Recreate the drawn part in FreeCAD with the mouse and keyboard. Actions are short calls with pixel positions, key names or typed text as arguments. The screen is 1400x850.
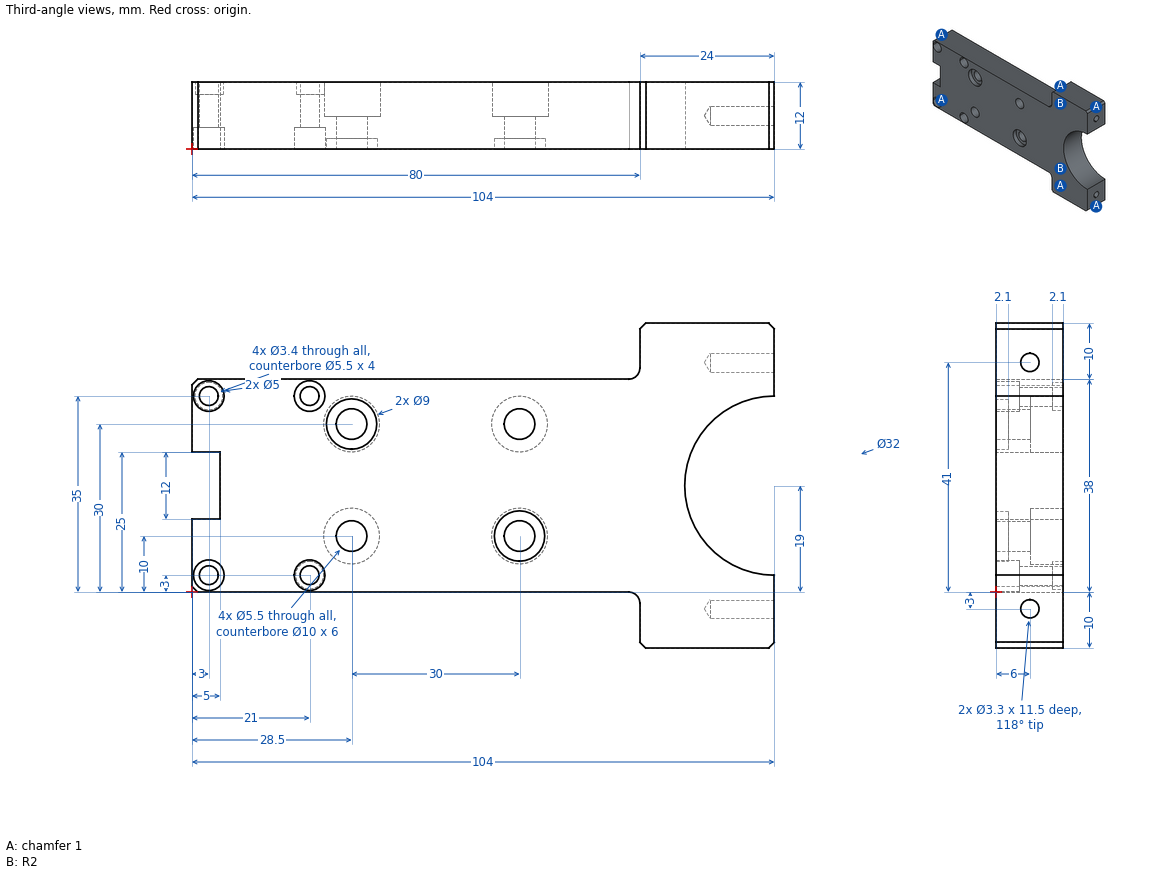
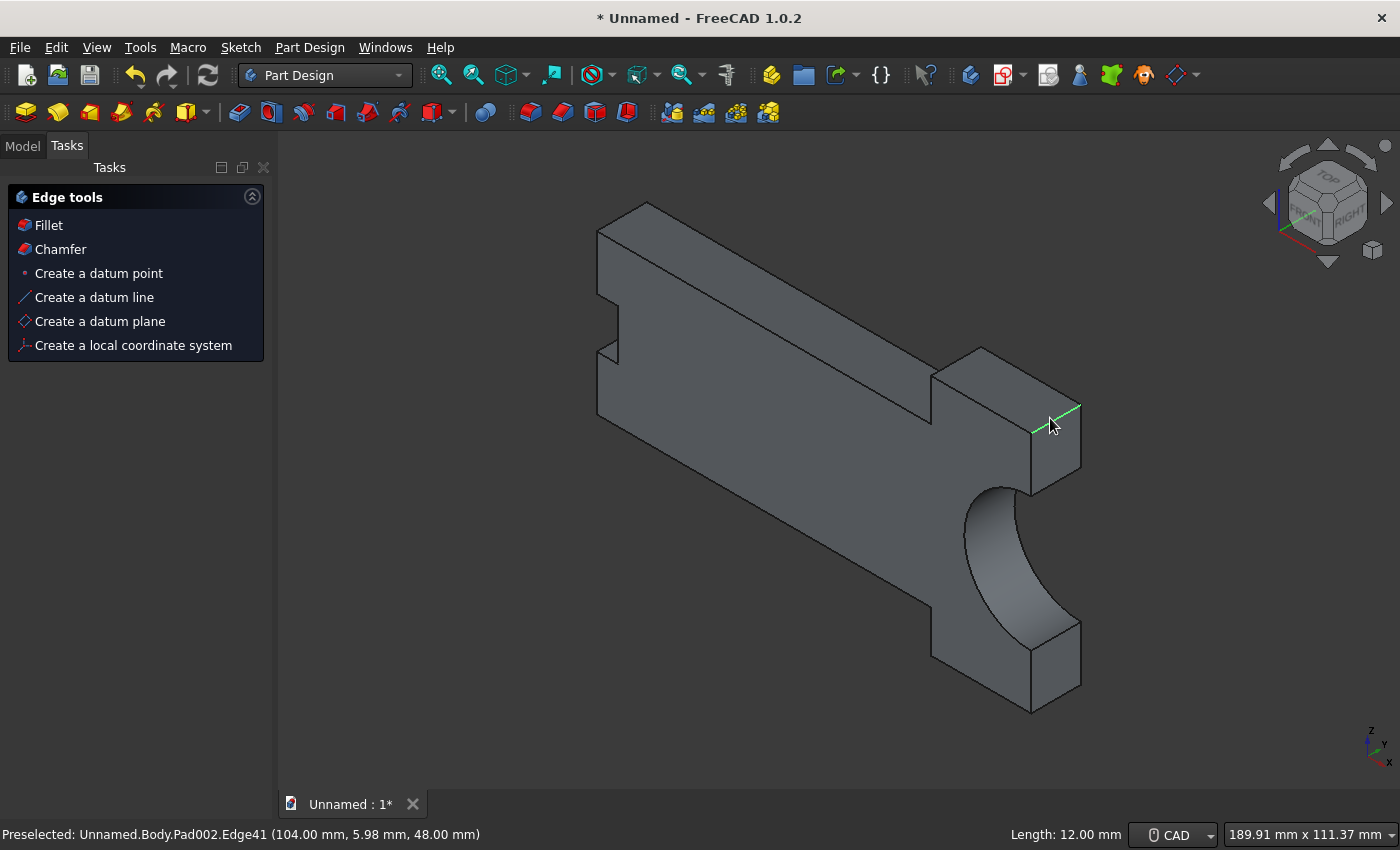
key(2)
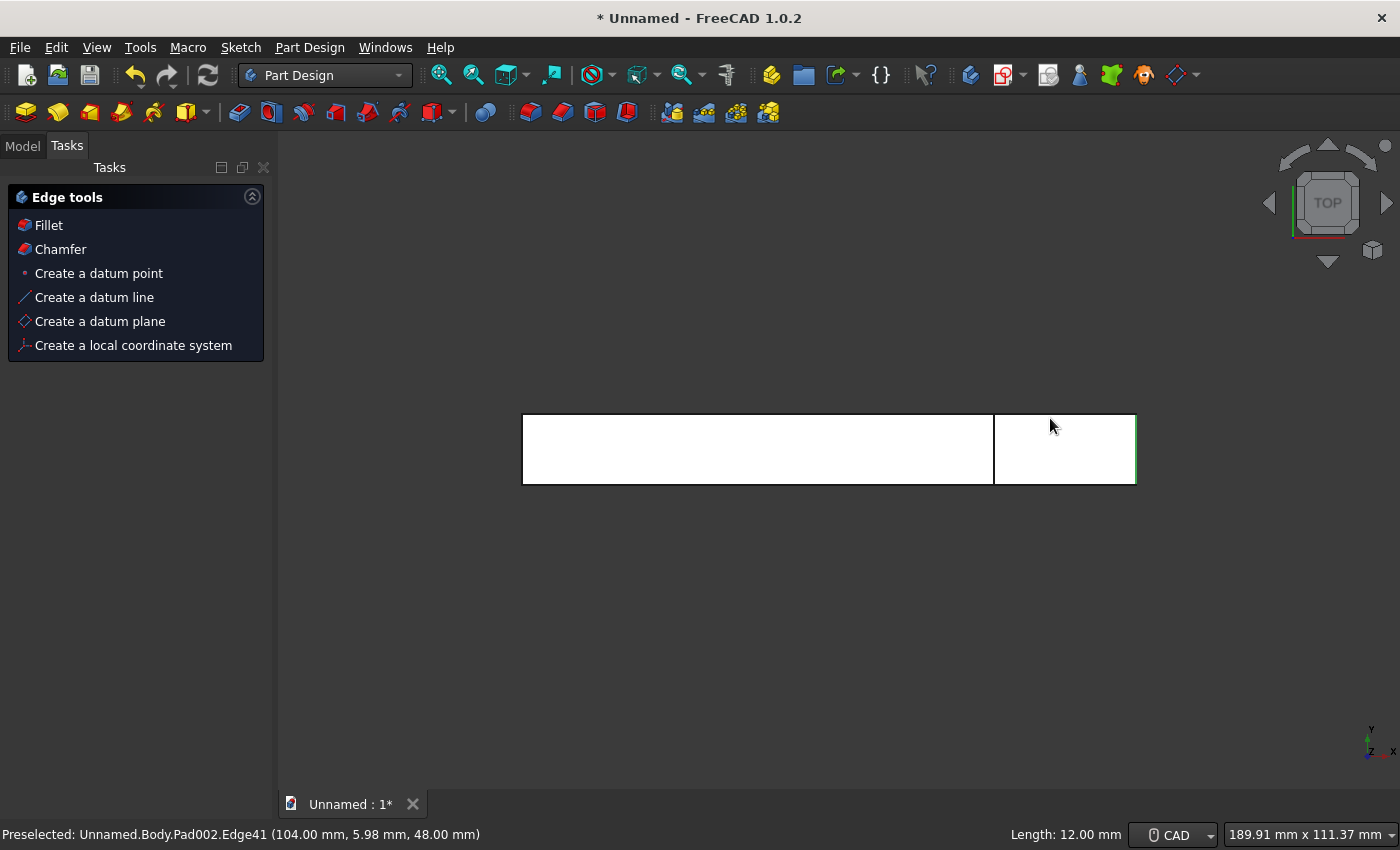
click(522, 449, ctrl)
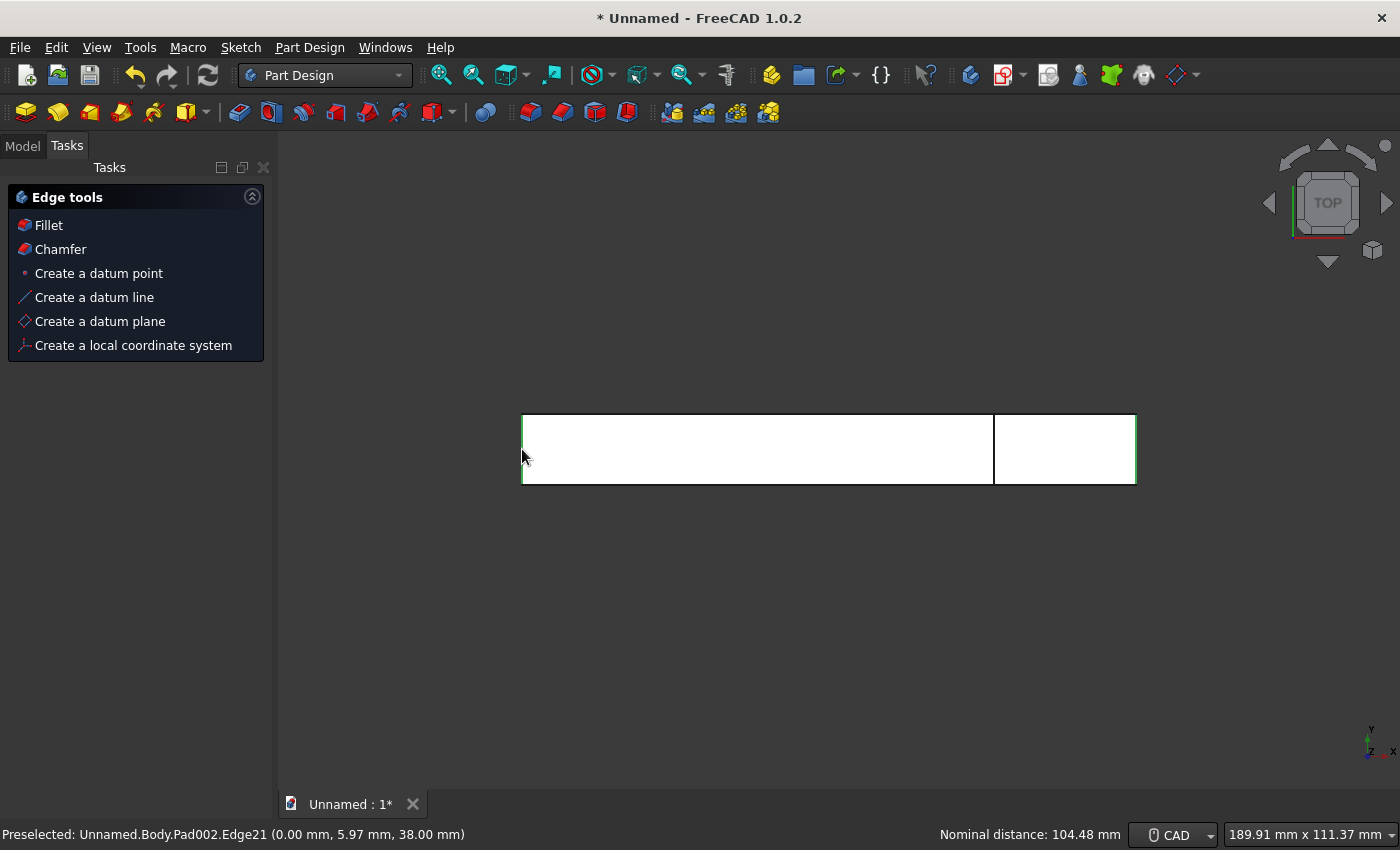
click(994, 449, ctrl)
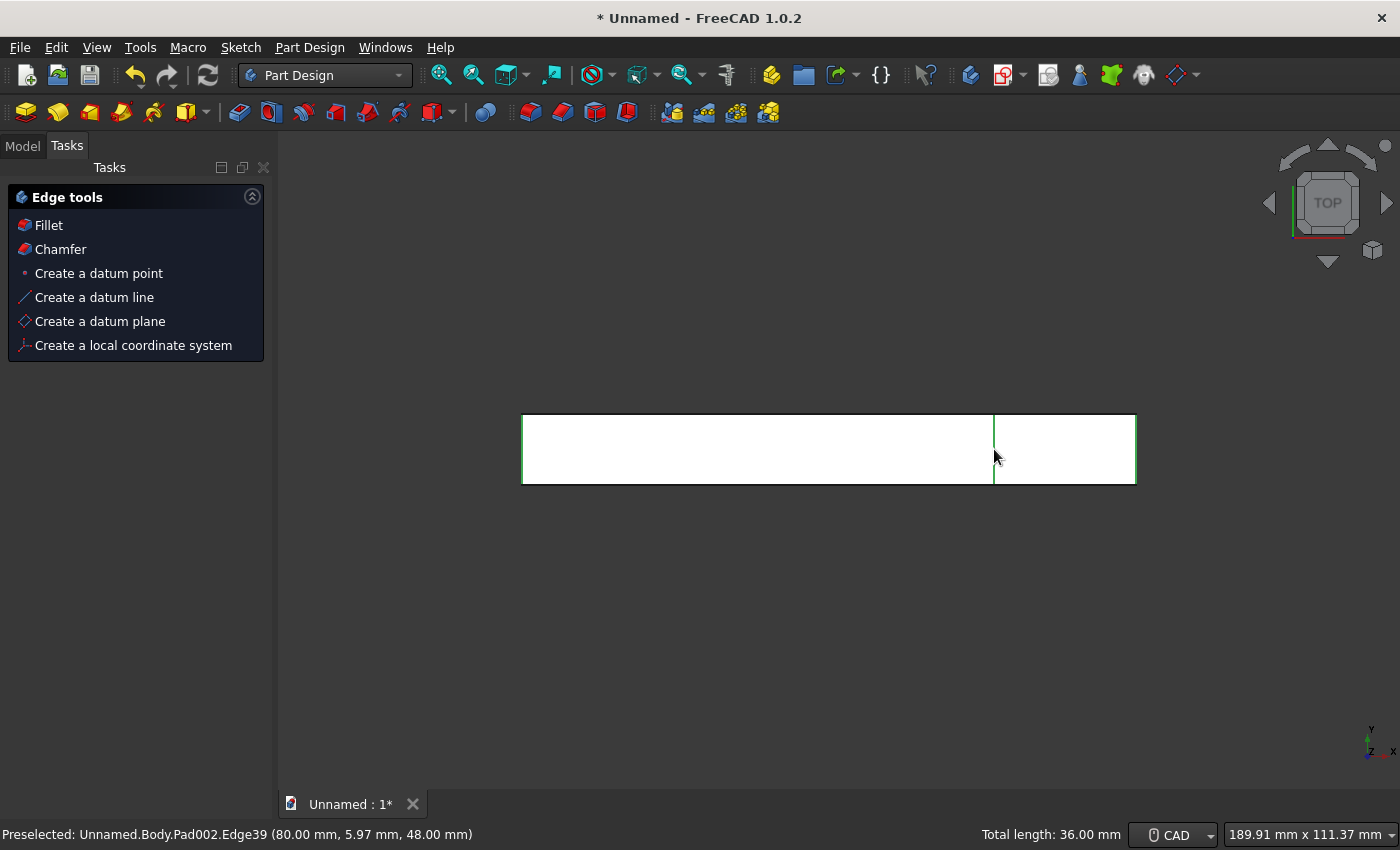
key(0)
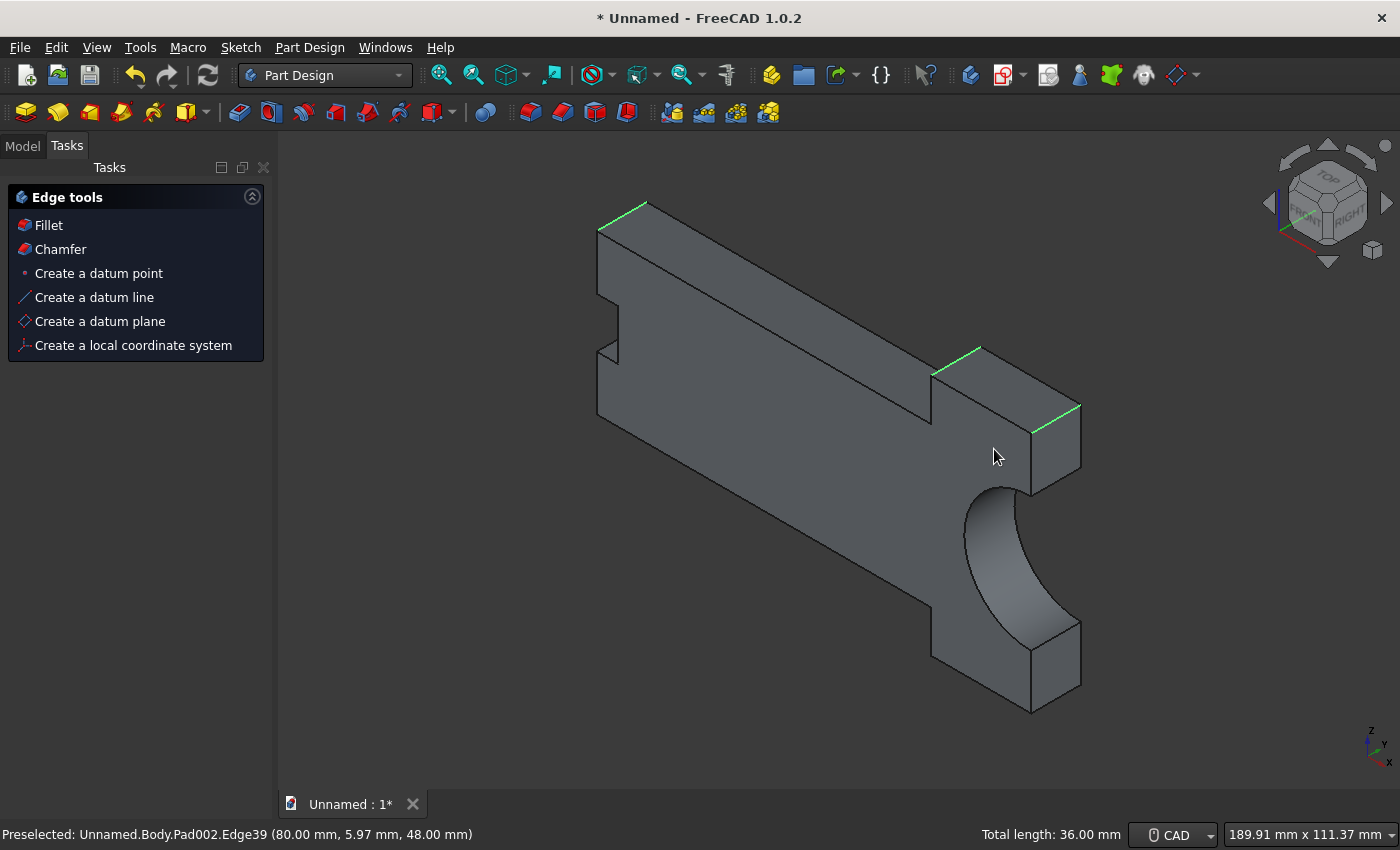
key(1)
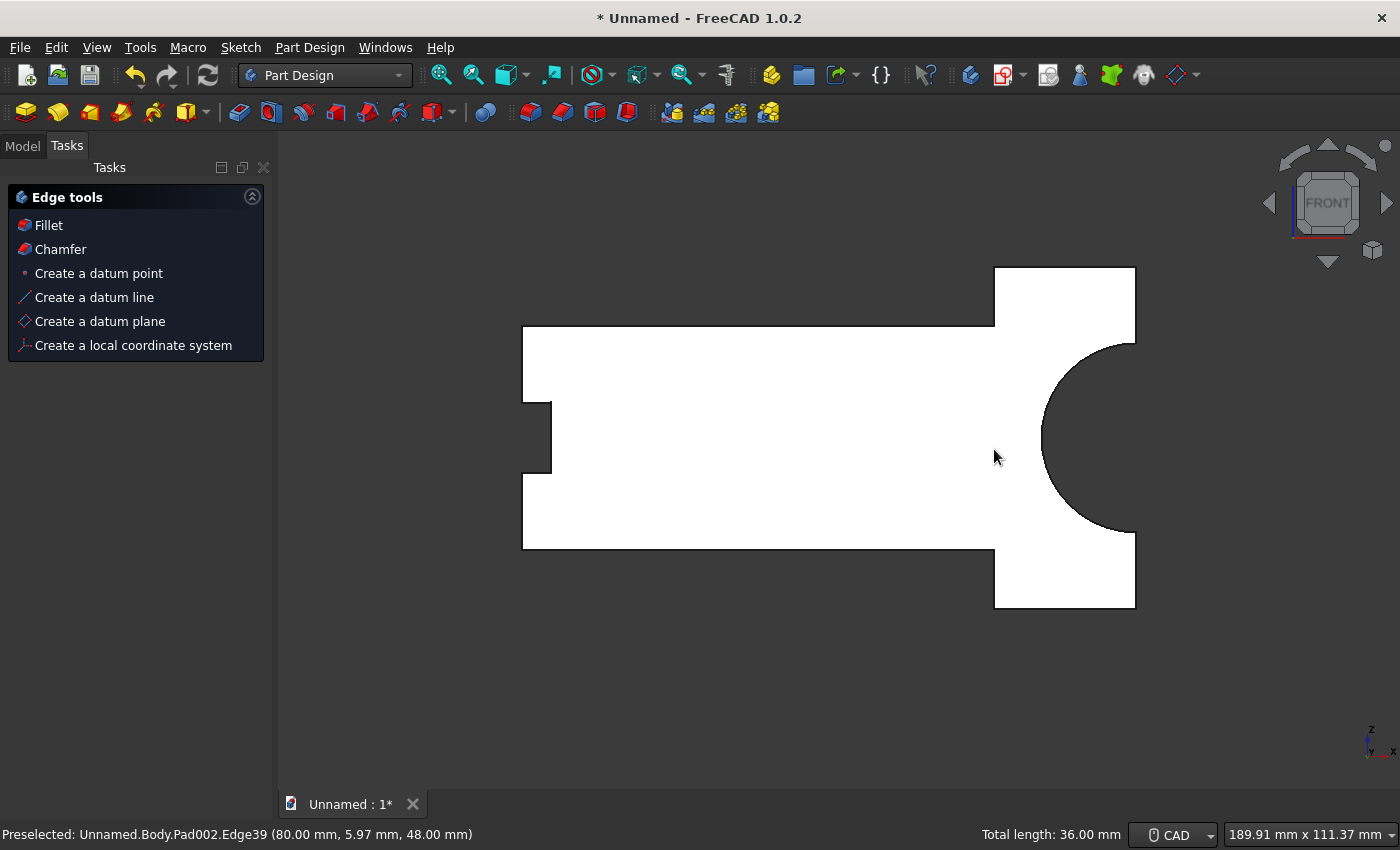
key(3)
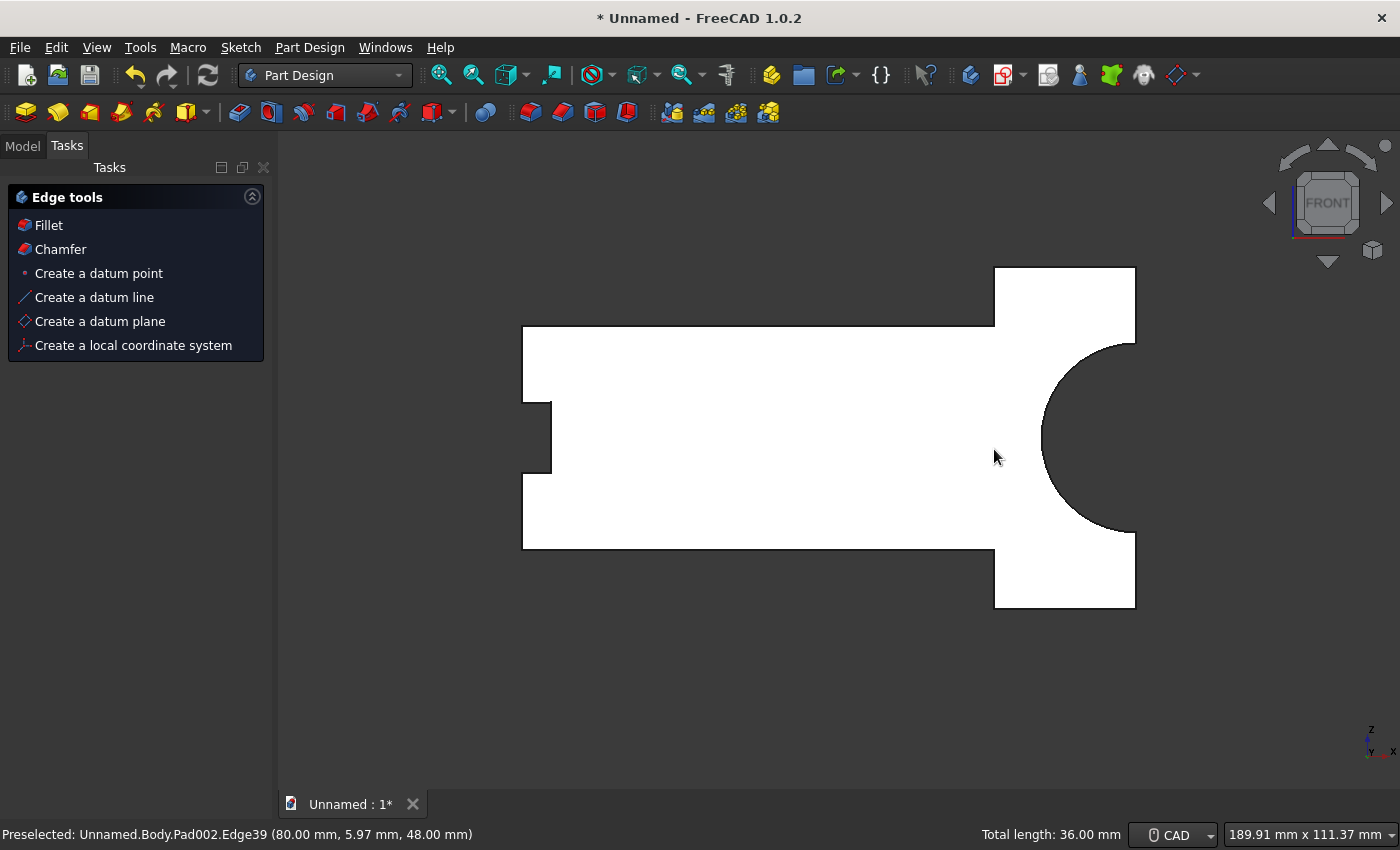
click(849, 608, ctrl)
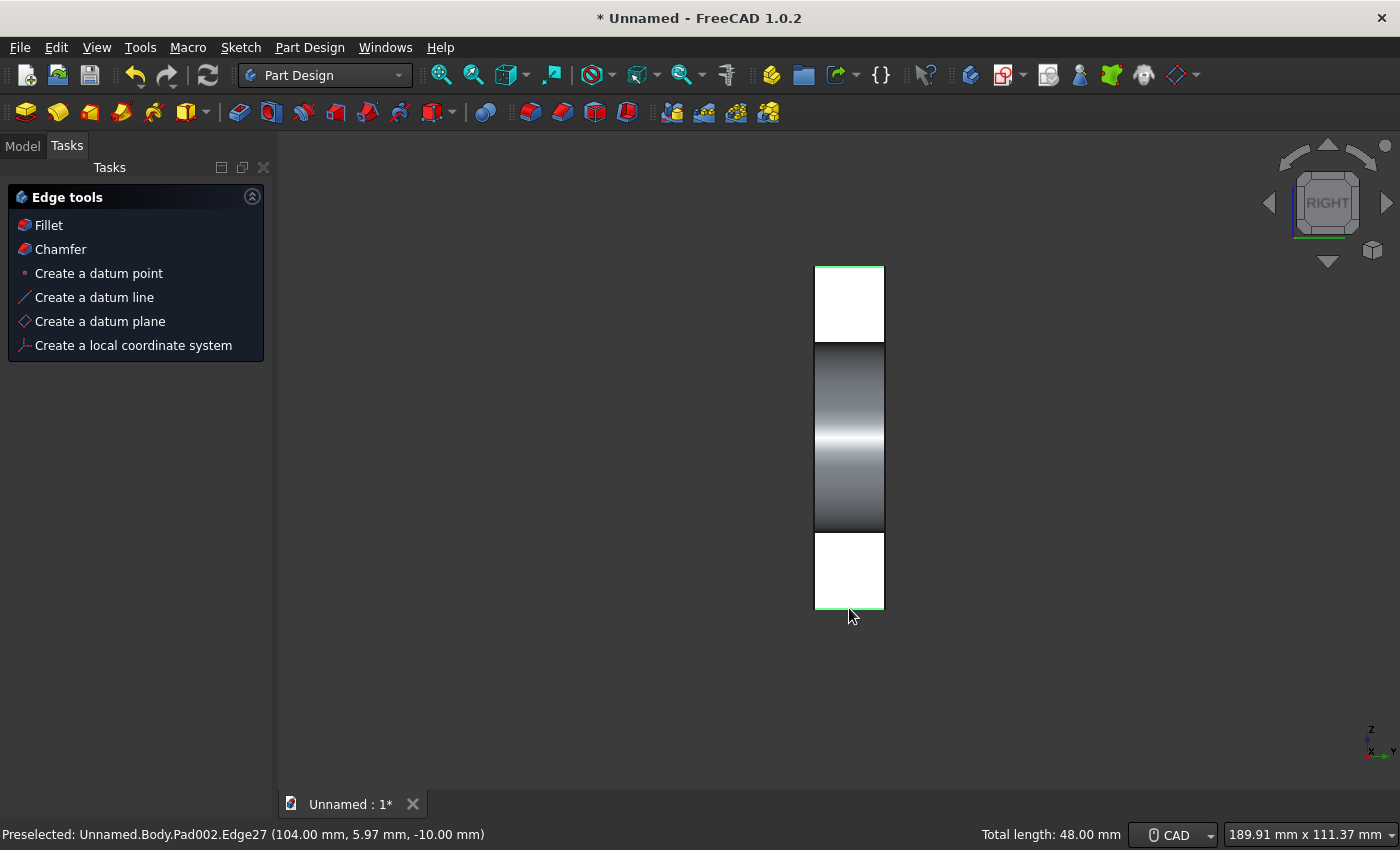
key(5)